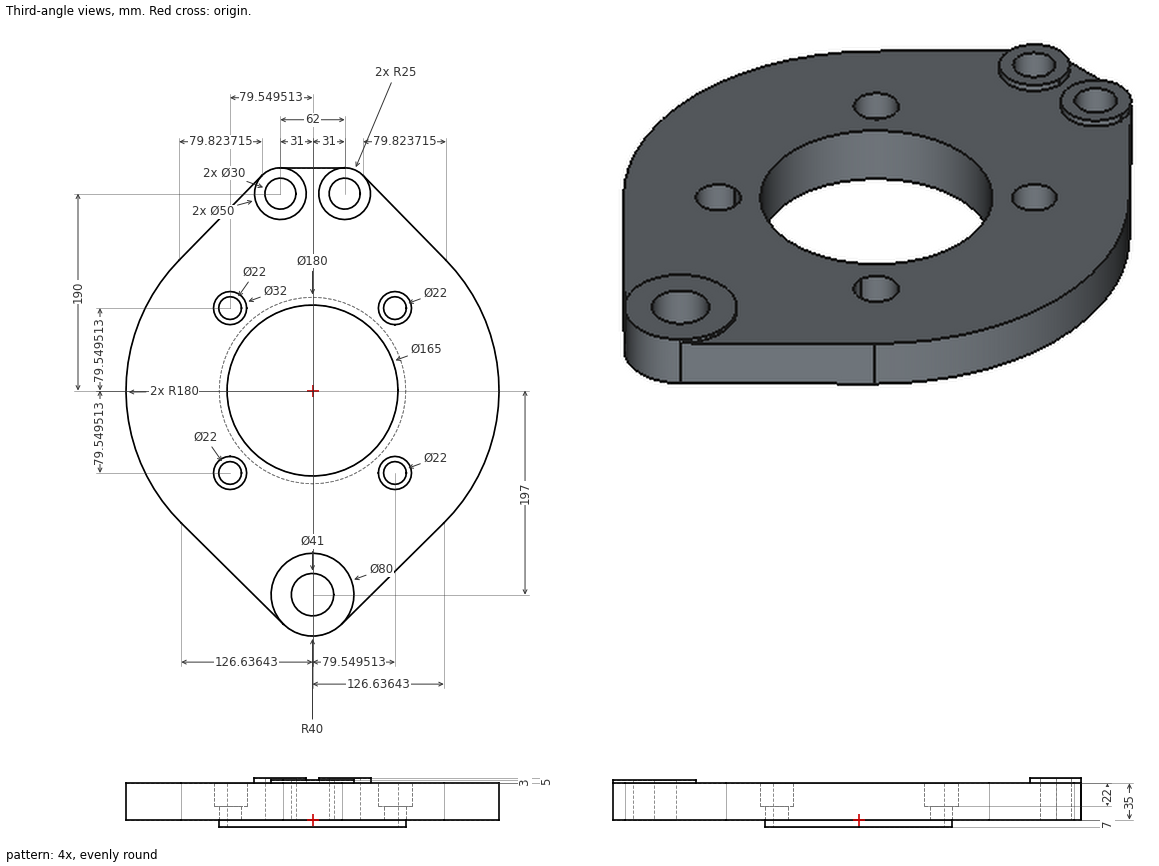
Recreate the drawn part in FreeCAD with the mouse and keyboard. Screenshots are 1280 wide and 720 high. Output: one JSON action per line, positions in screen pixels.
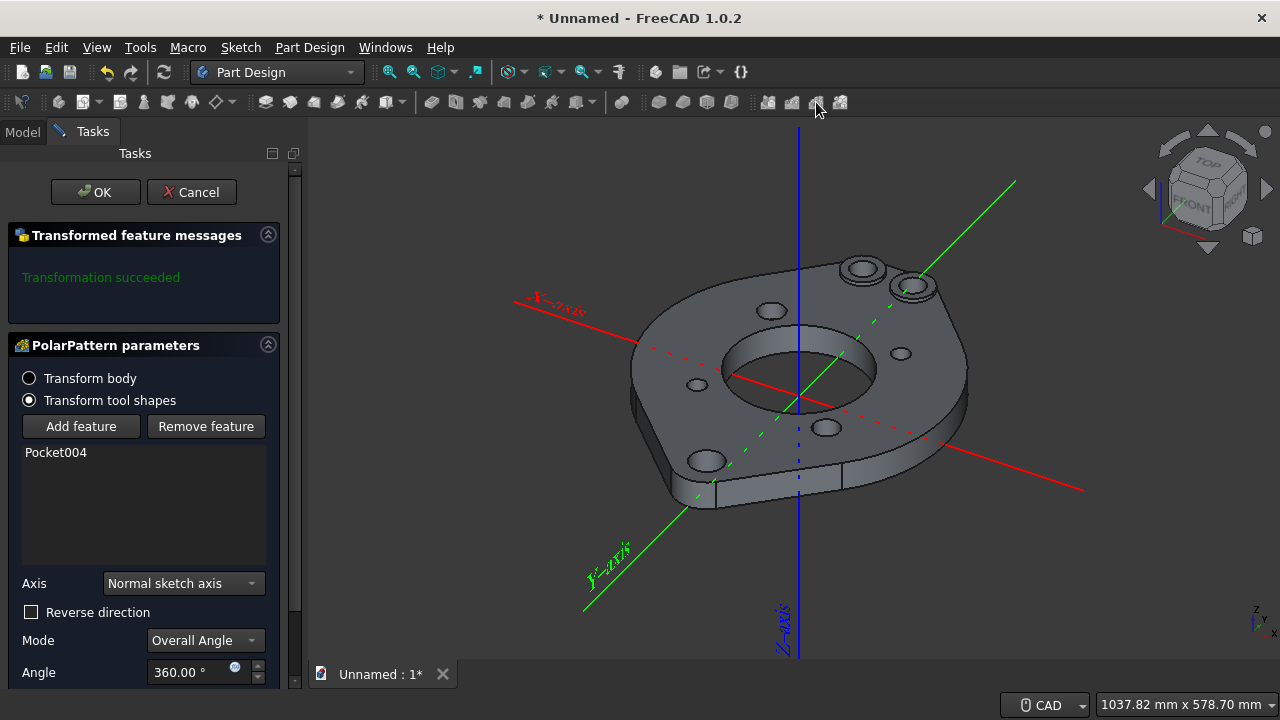
{"action": "left_click", "coordinate": [184, 584]}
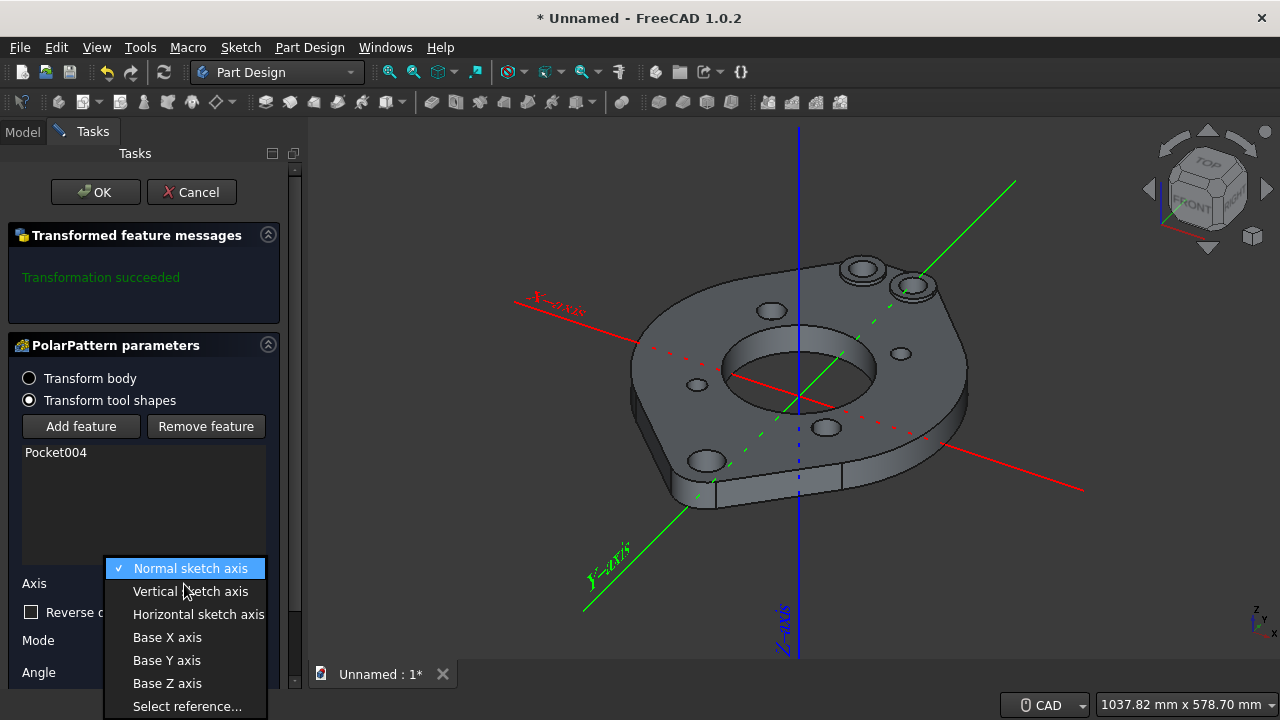
{"action": "left_click", "coordinate": [184, 684]}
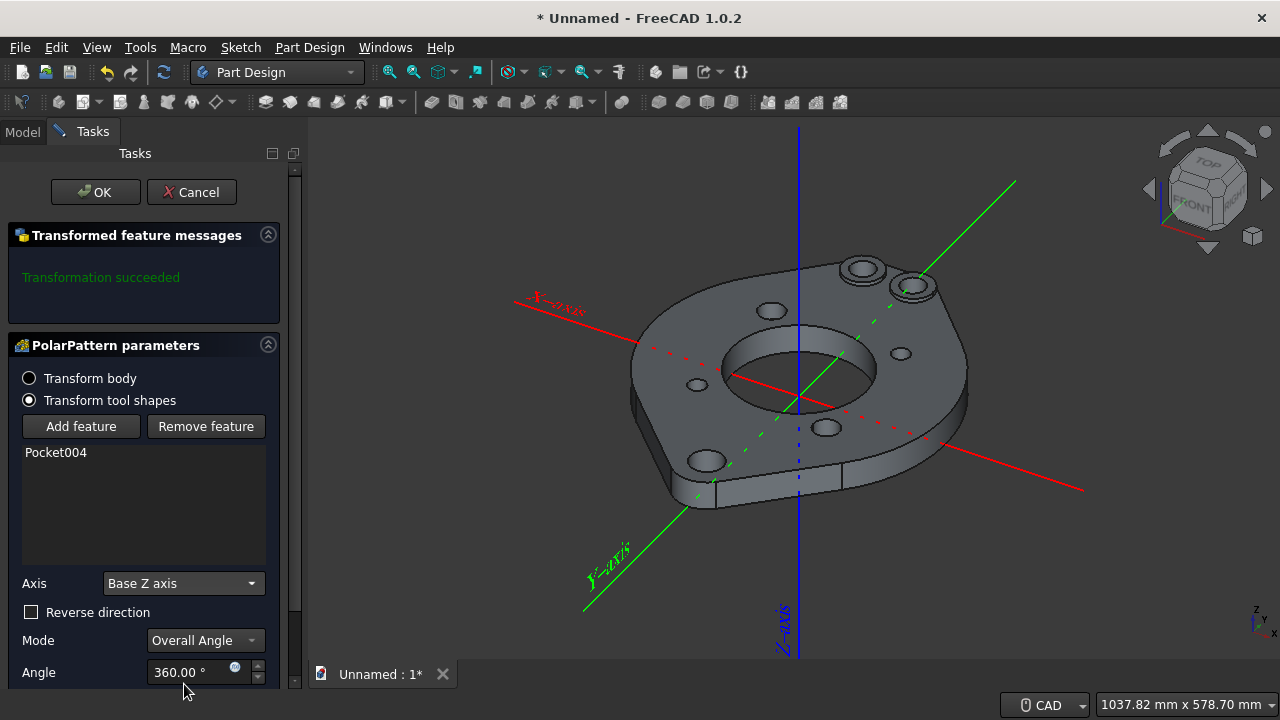
{"action": "scroll", "coordinate": [295, 426], "scroll_direction": "down", "scroll_amount": 2}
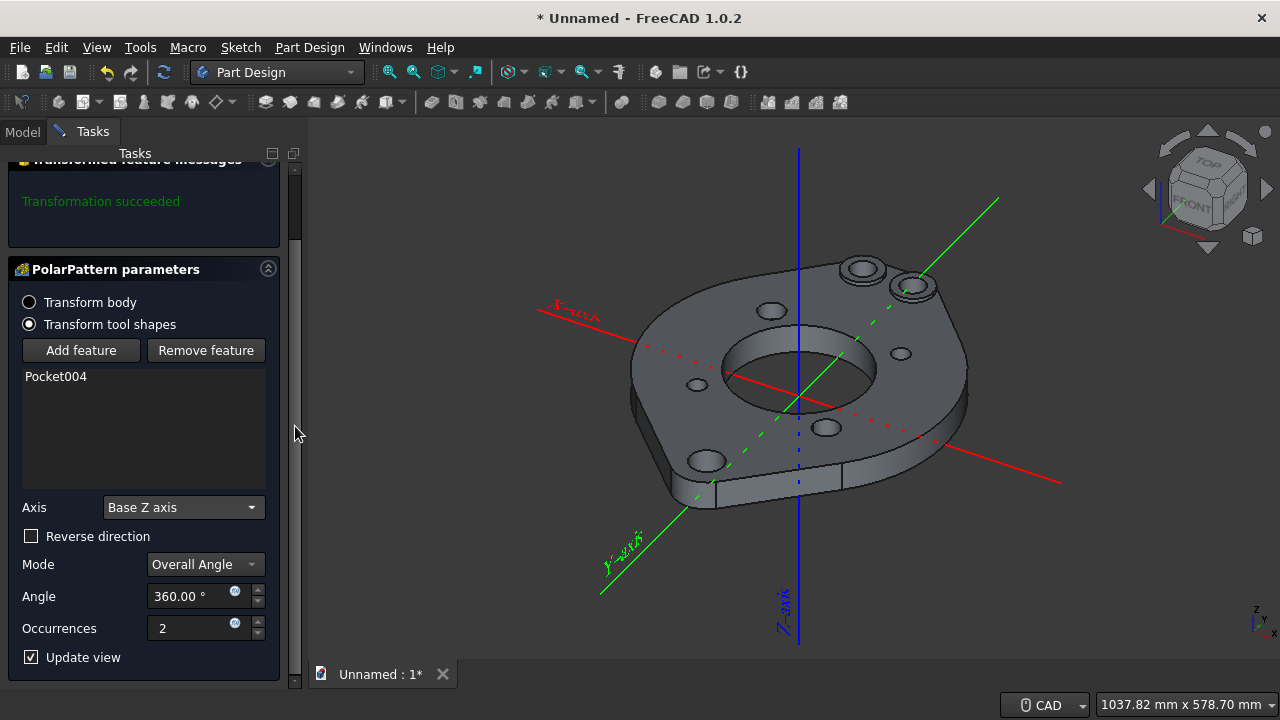
{"action": "triple_click", "coordinate": [198, 628]}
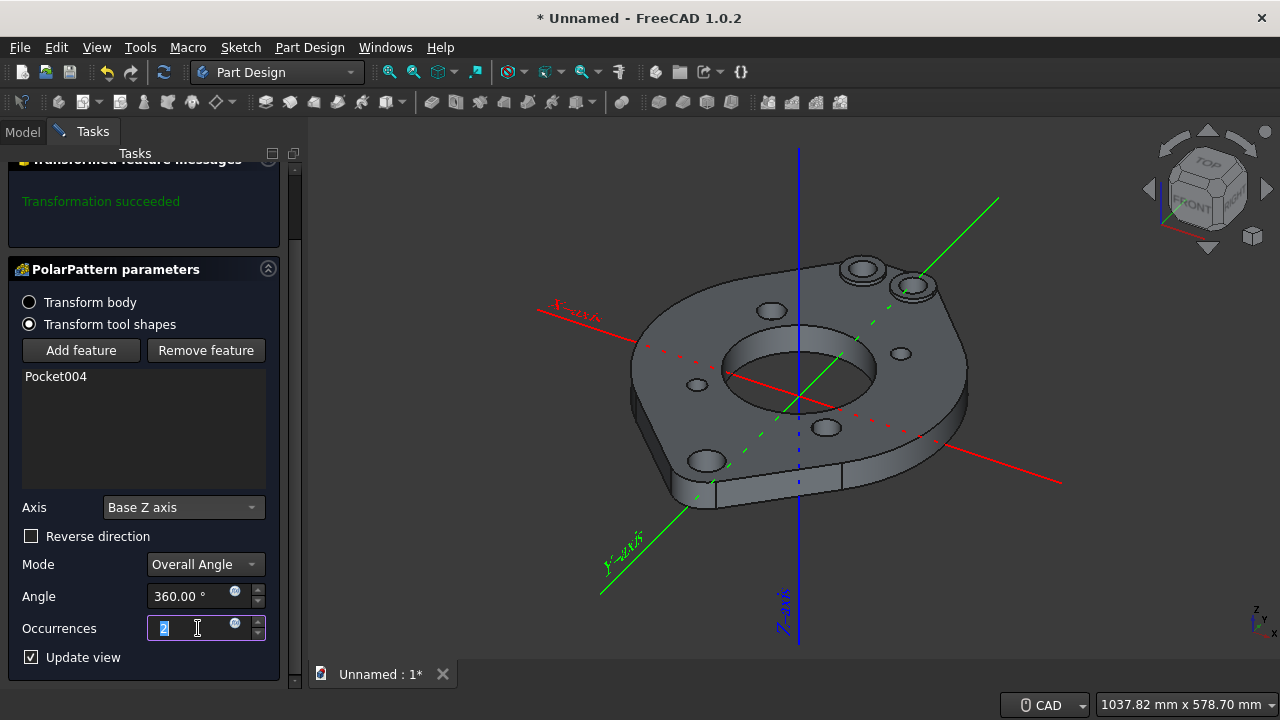
{"action": "type", "text": "4"}
{"action": "key", "text": "Tab"}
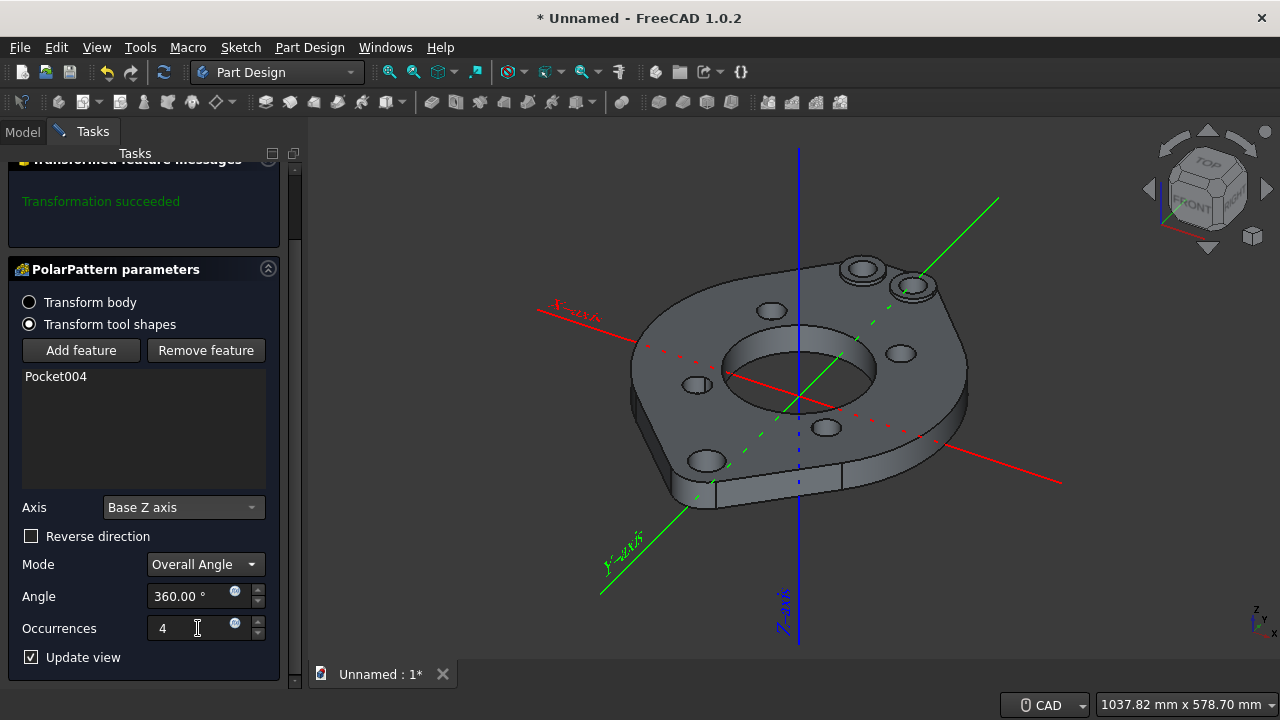
{"action": "scroll", "coordinate": [295, 426], "scroll_direction": "up", "scroll_amount": 3}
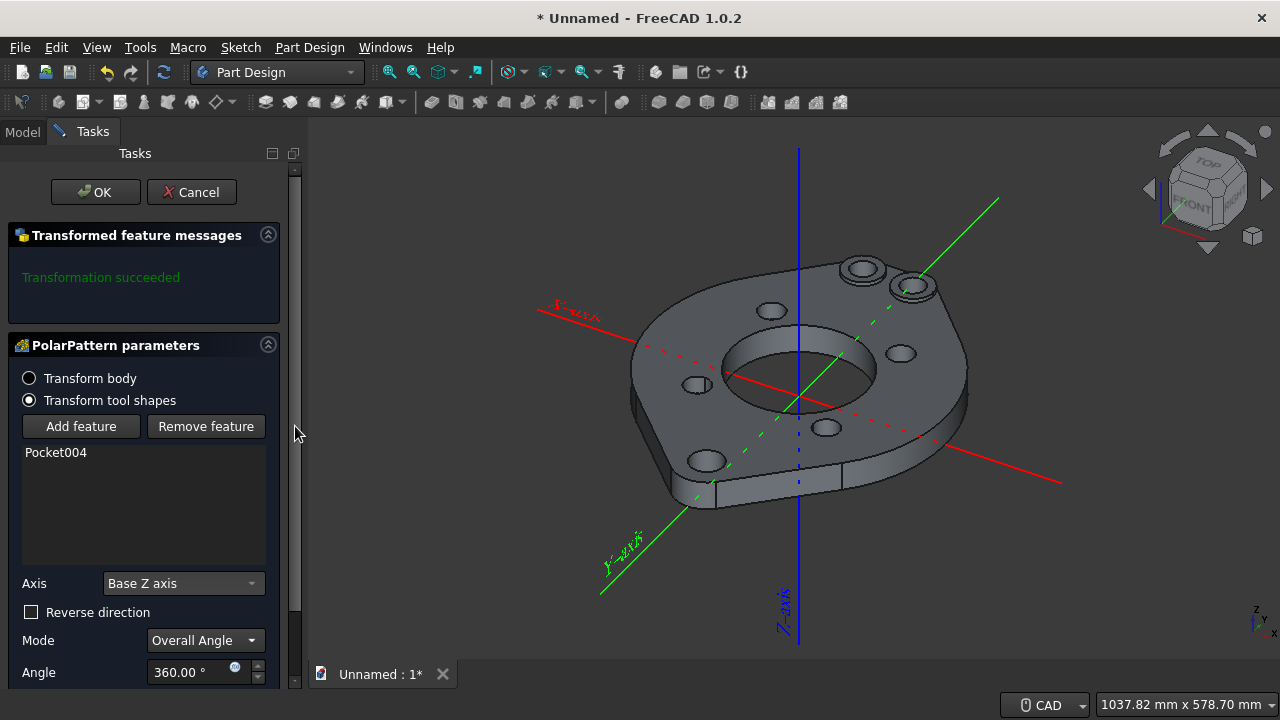
{"action": "left_click", "coordinate": [96, 192]}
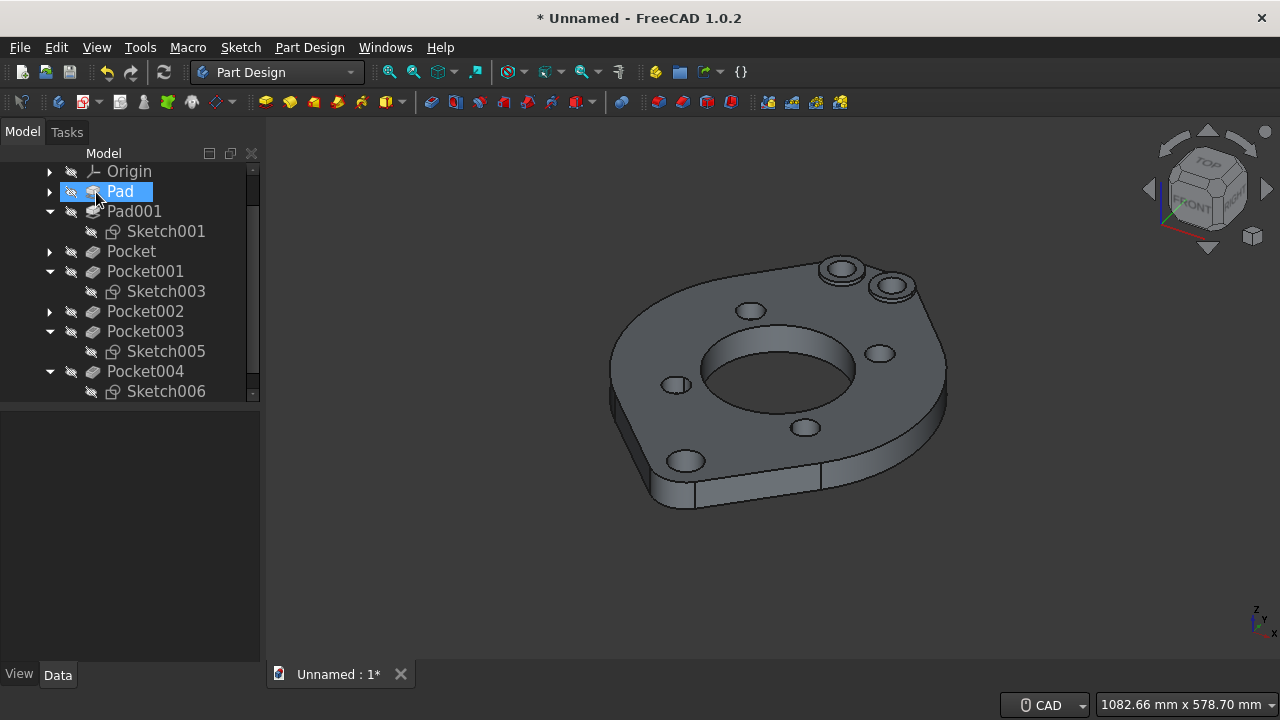
{"action": "left_click", "coordinate": [671, 420]}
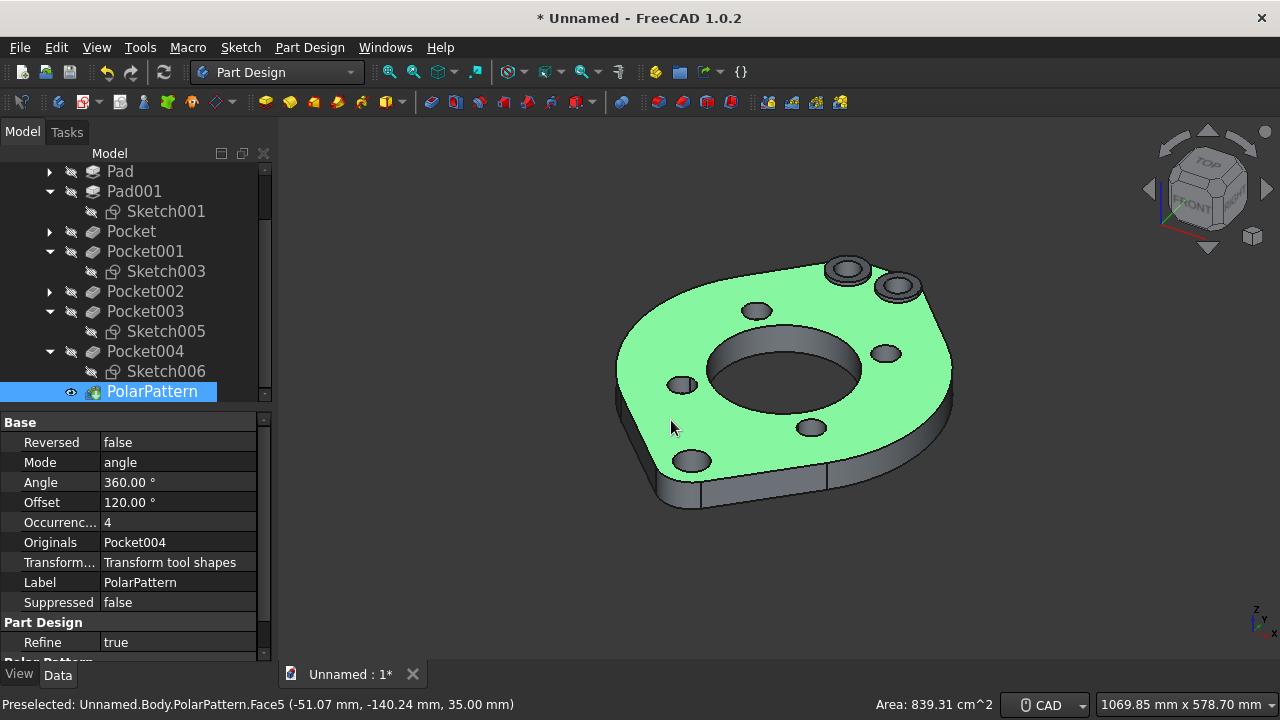
{"action": "left_click", "coordinate": [84, 102]}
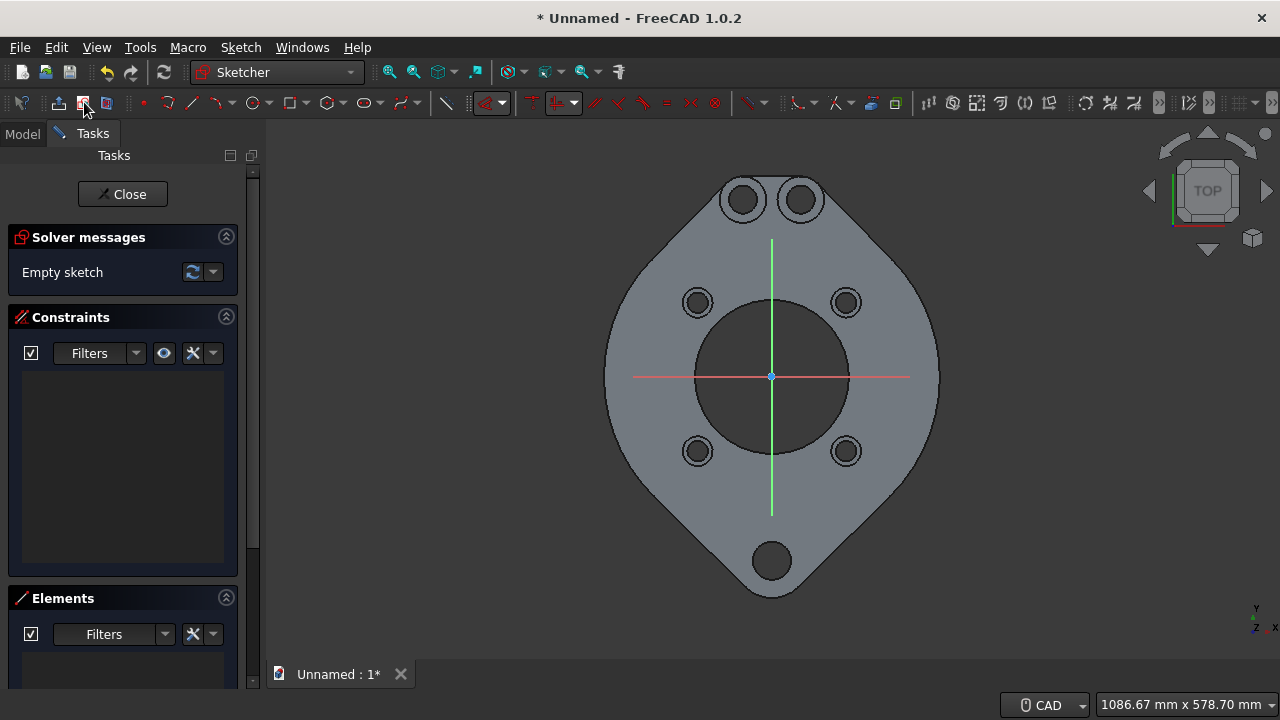
{"action": "key", "text": "q s"}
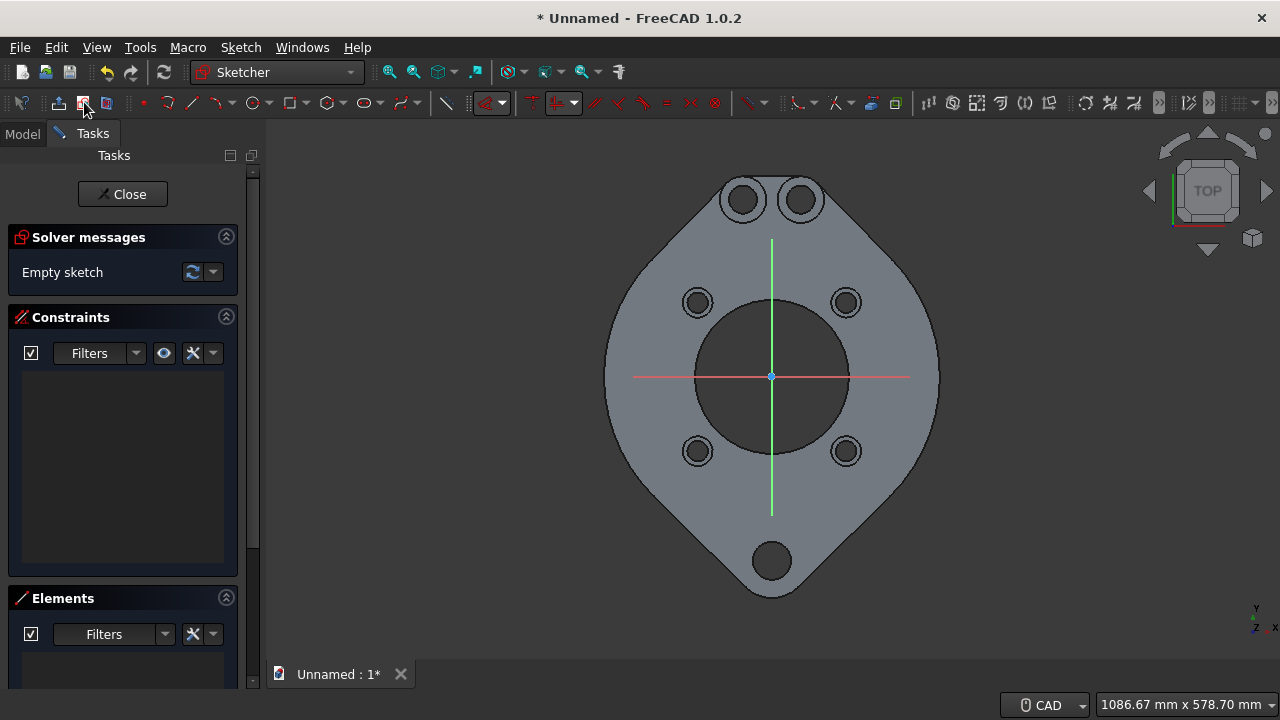
{"action": "scroll", "coordinate": [789, 604], "scroll_direction": "up", "scroll_amount": 8}